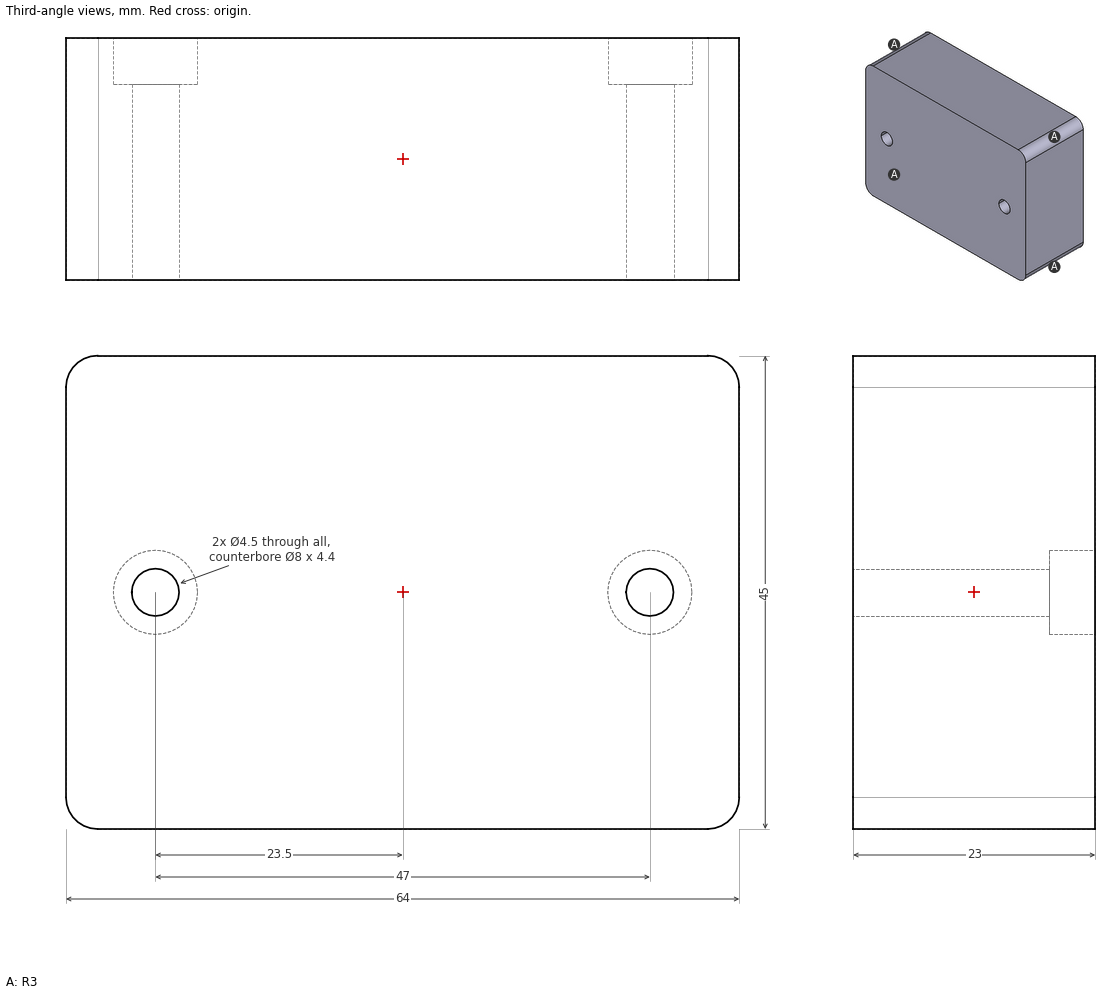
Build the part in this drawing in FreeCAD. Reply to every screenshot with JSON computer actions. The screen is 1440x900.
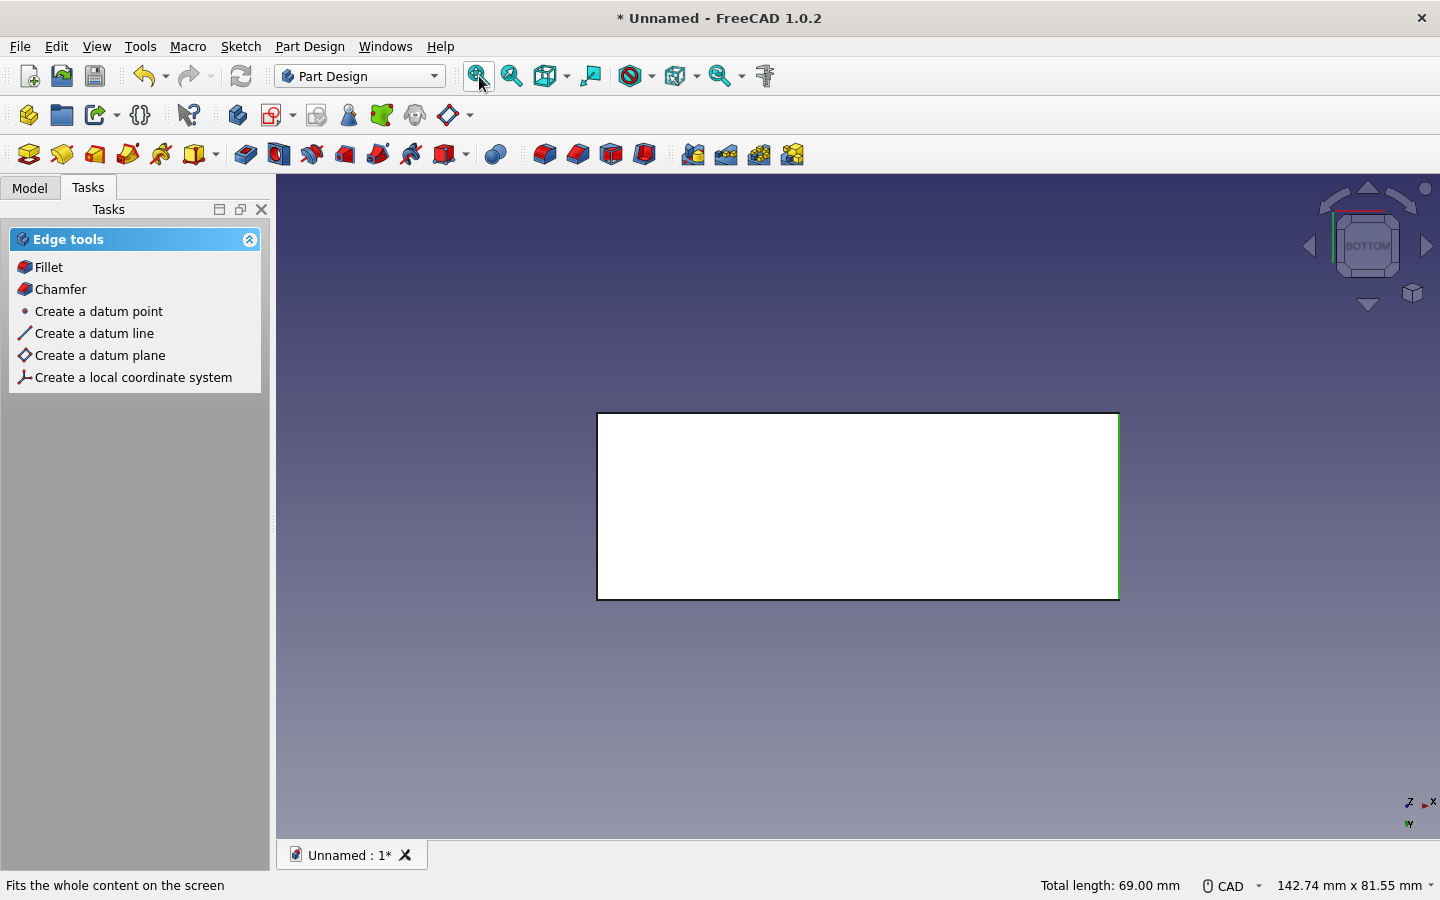
{"action": "left_click", "coordinate": [597, 505], "text": "ctrl"}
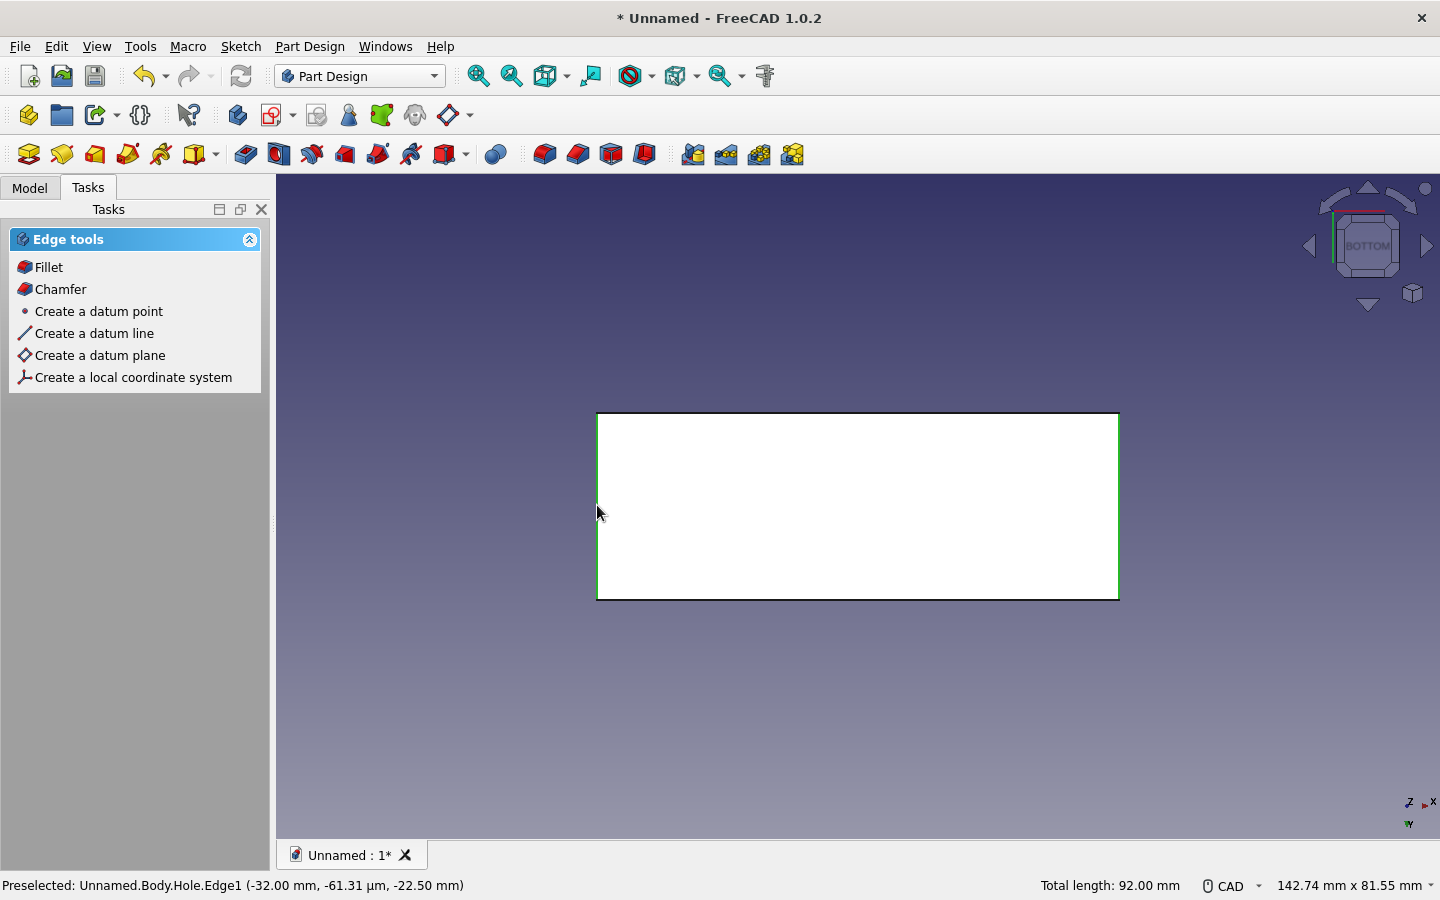
{"action": "left_click", "coordinate": [545, 154]}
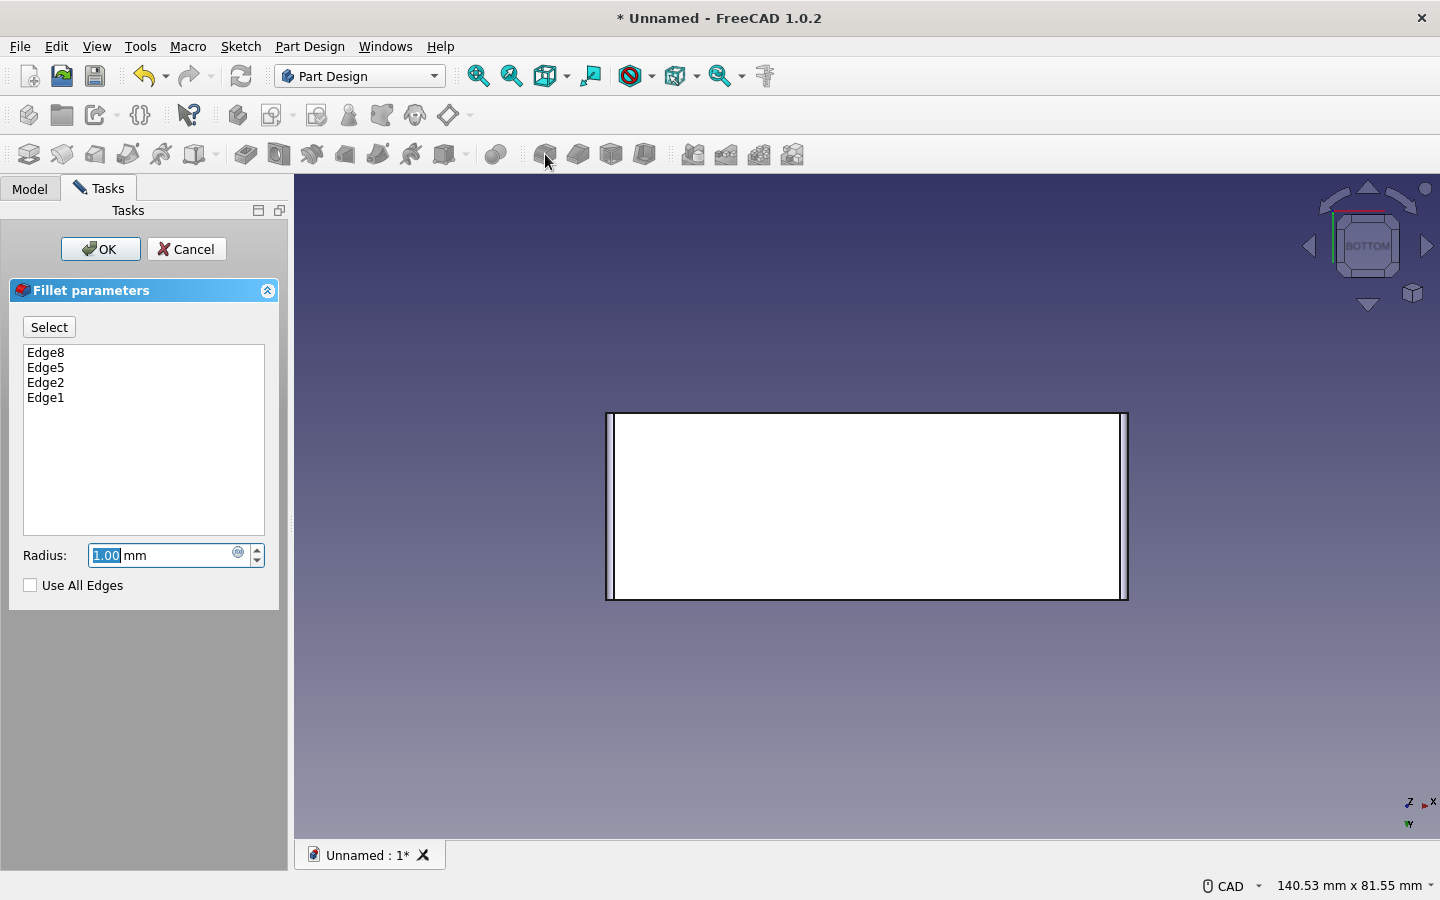
{"action": "type", "text": "3"}
{"action": "key", "text": "Tab"}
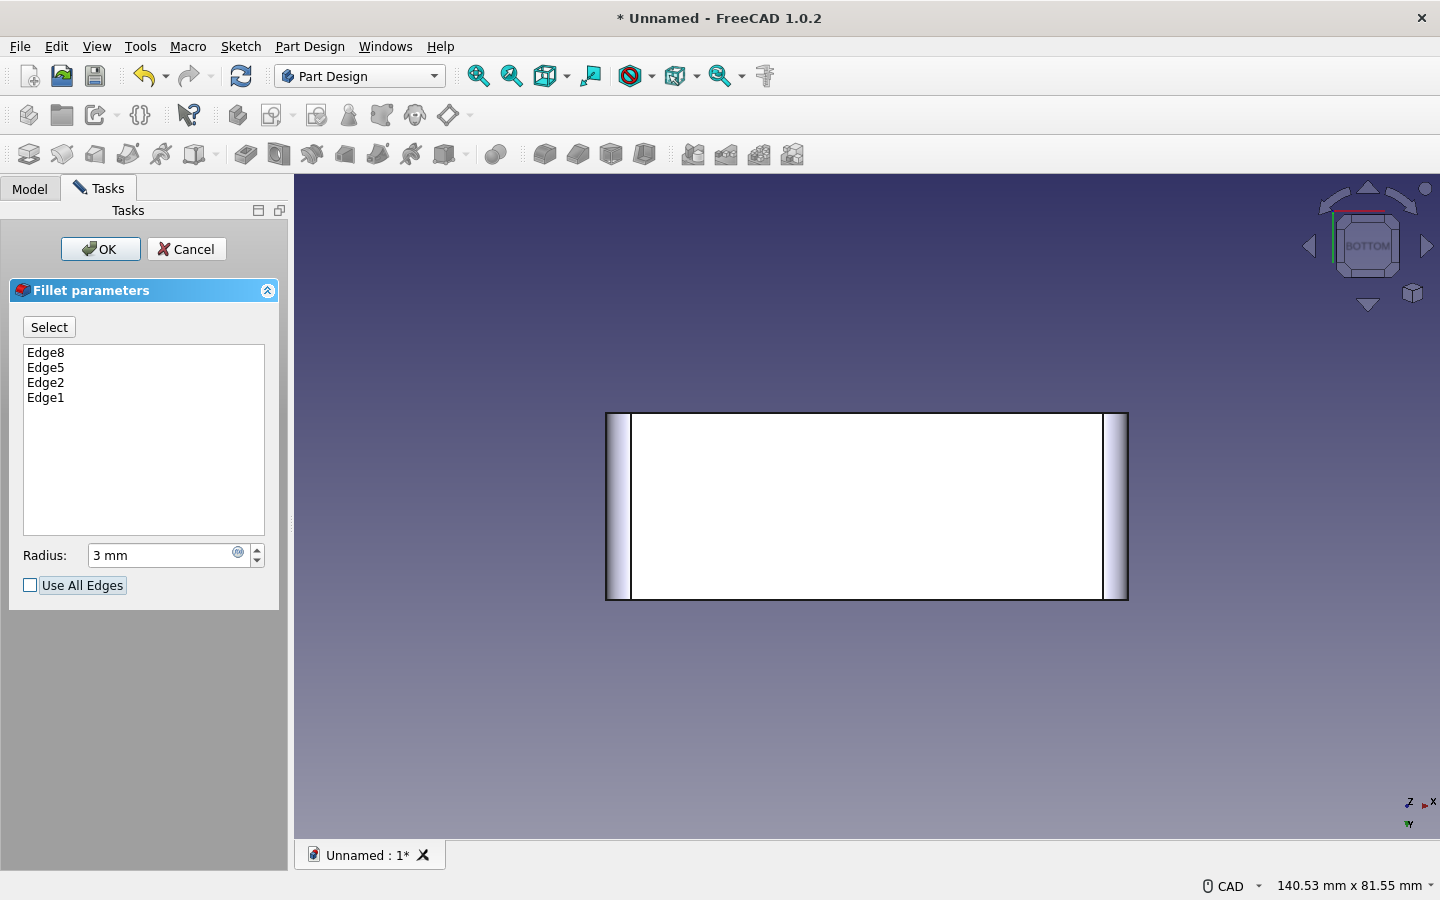
{"action": "left_click", "coordinate": [101, 249]}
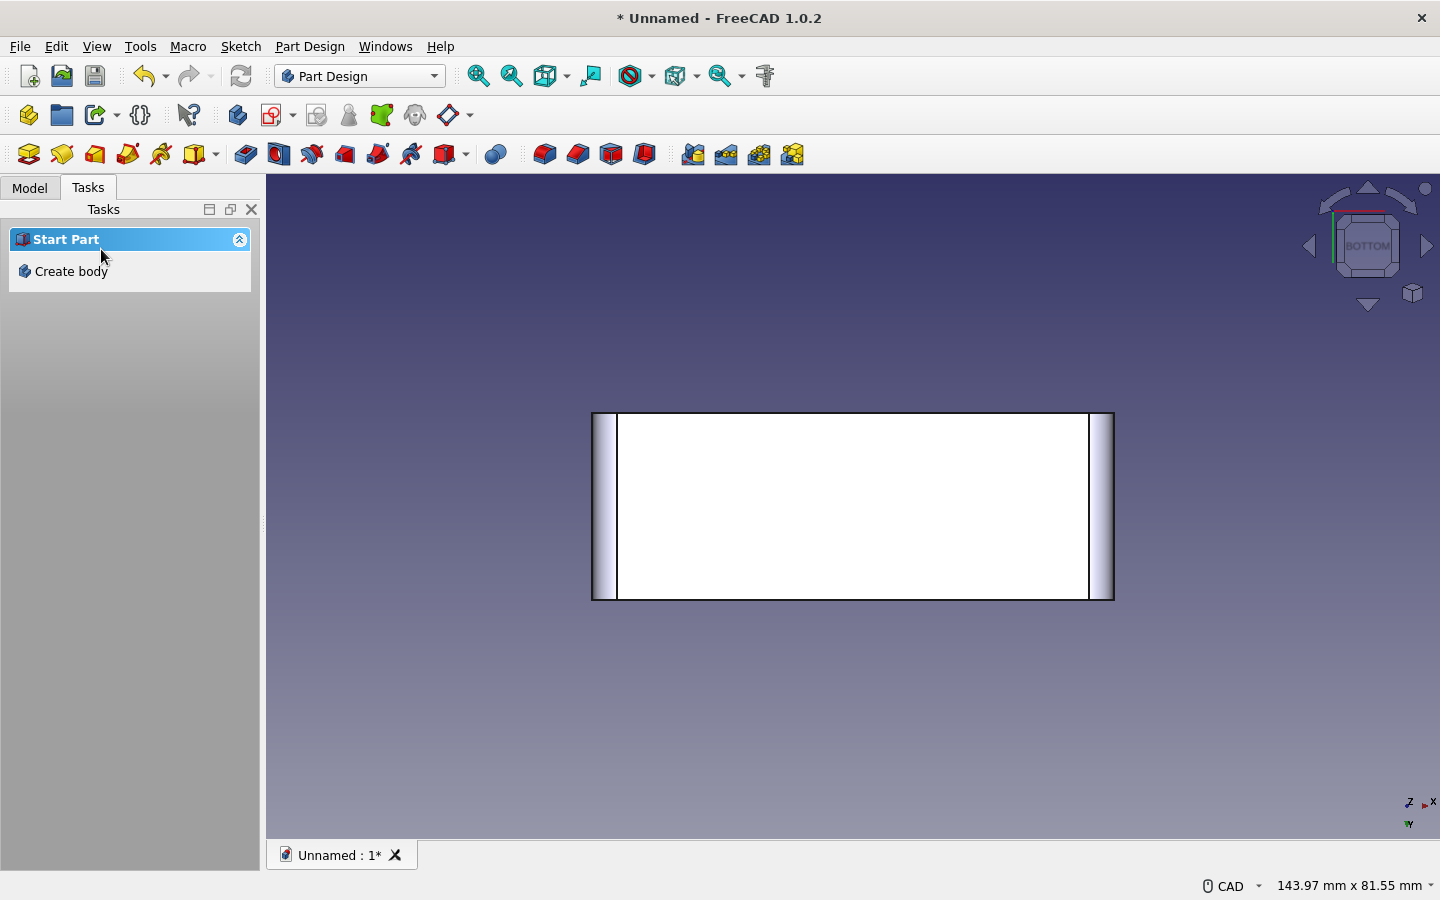
{"action": "key", "text": "0"}